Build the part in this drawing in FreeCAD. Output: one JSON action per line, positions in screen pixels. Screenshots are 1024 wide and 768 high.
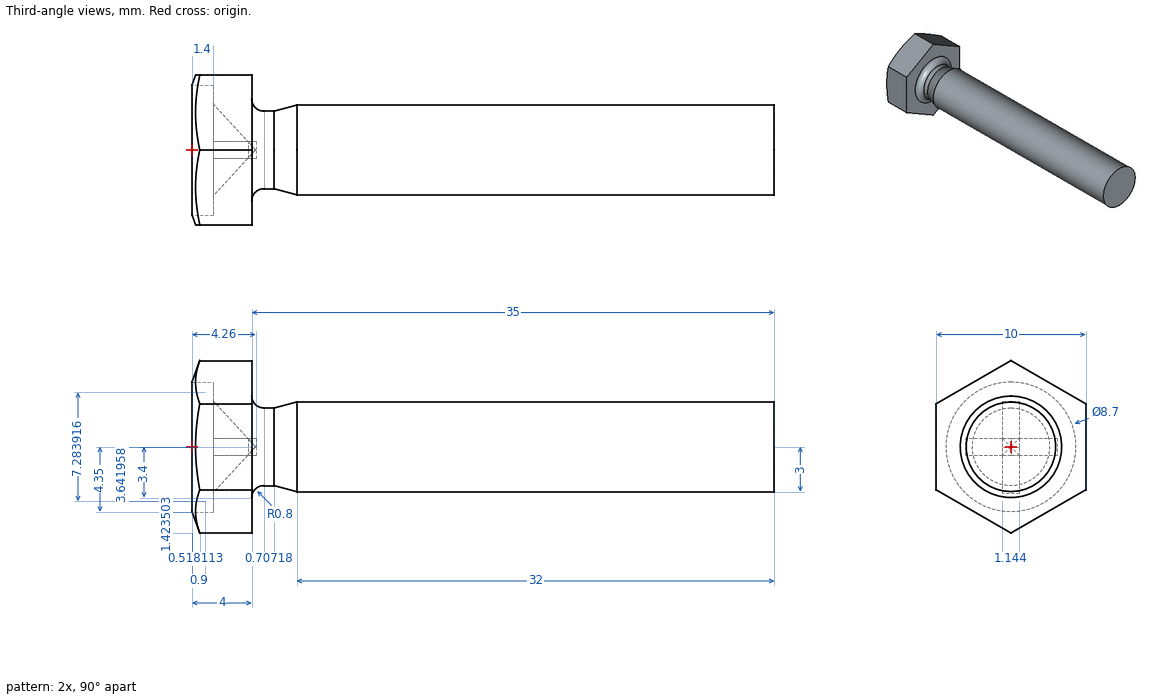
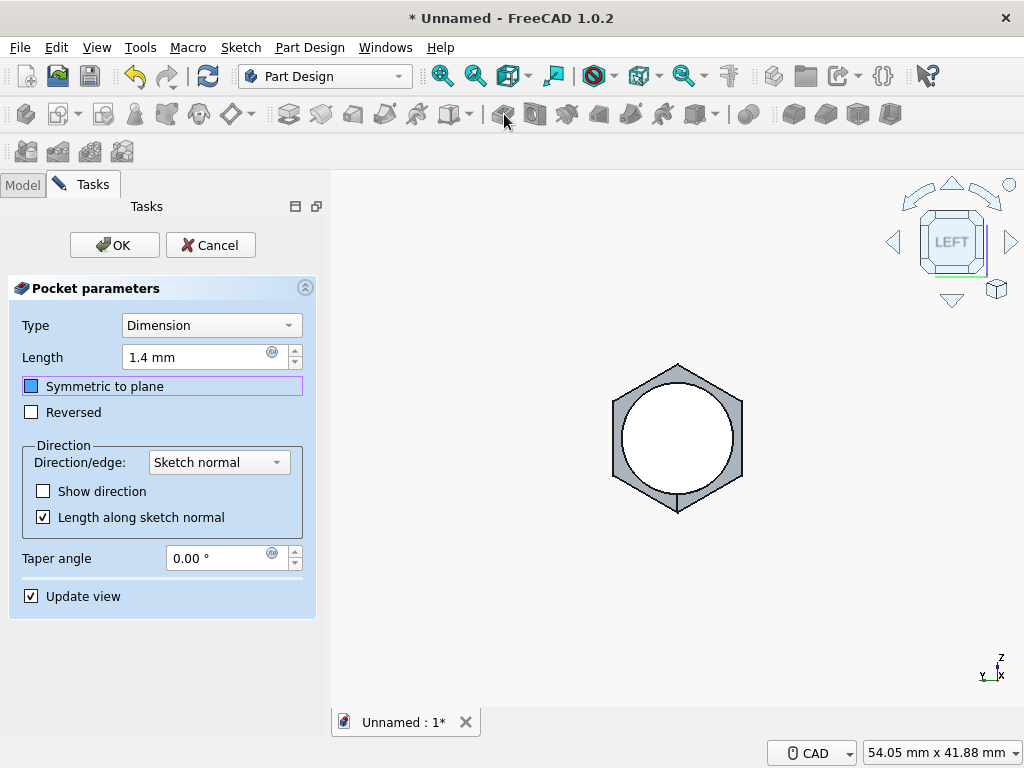
{"action": "left_click", "coordinate": [115, 245]}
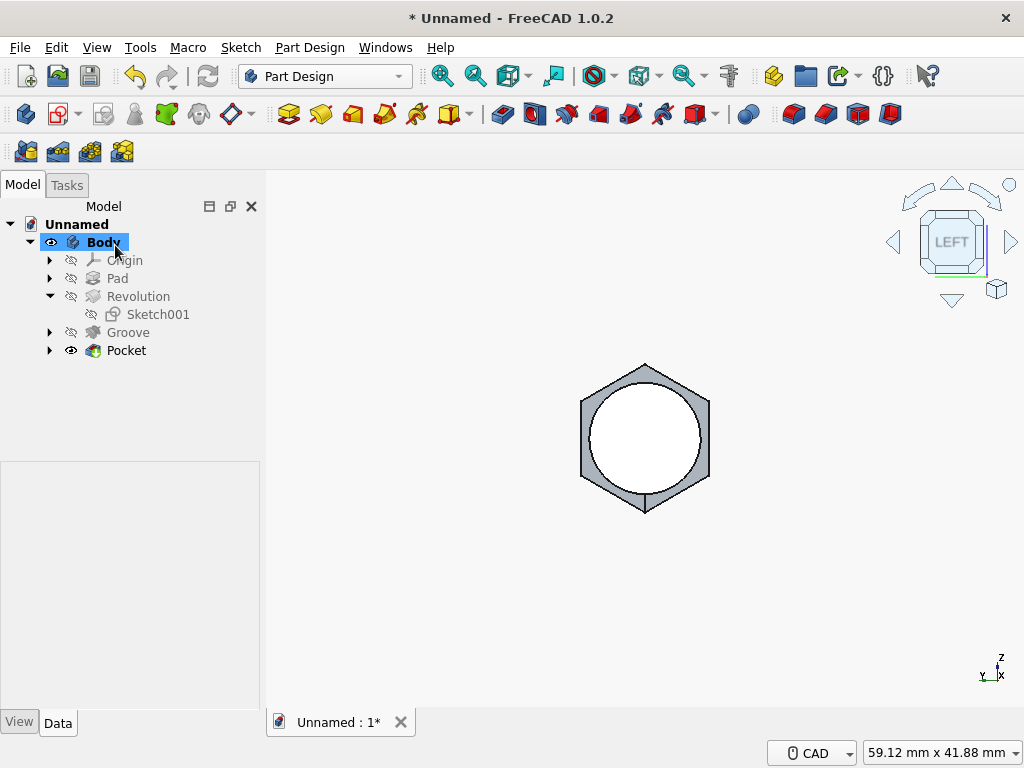
{"action": "left_click", "coordinate": [444, 76]}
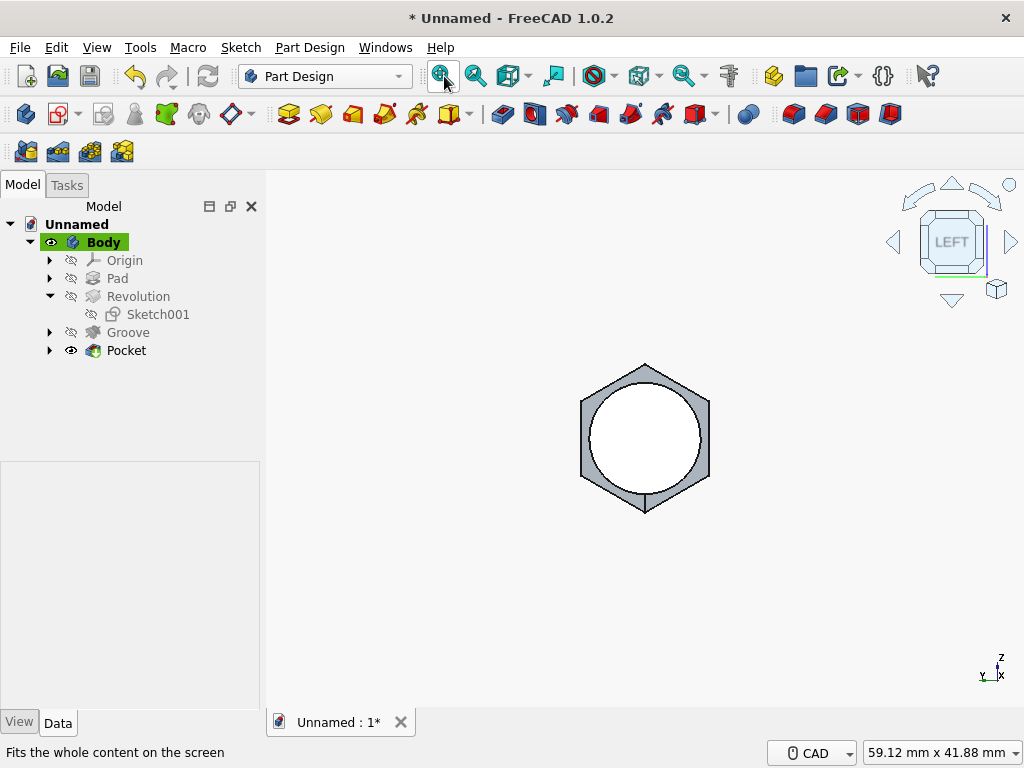
{"action": "left_click", "coordinate": [58, 114]}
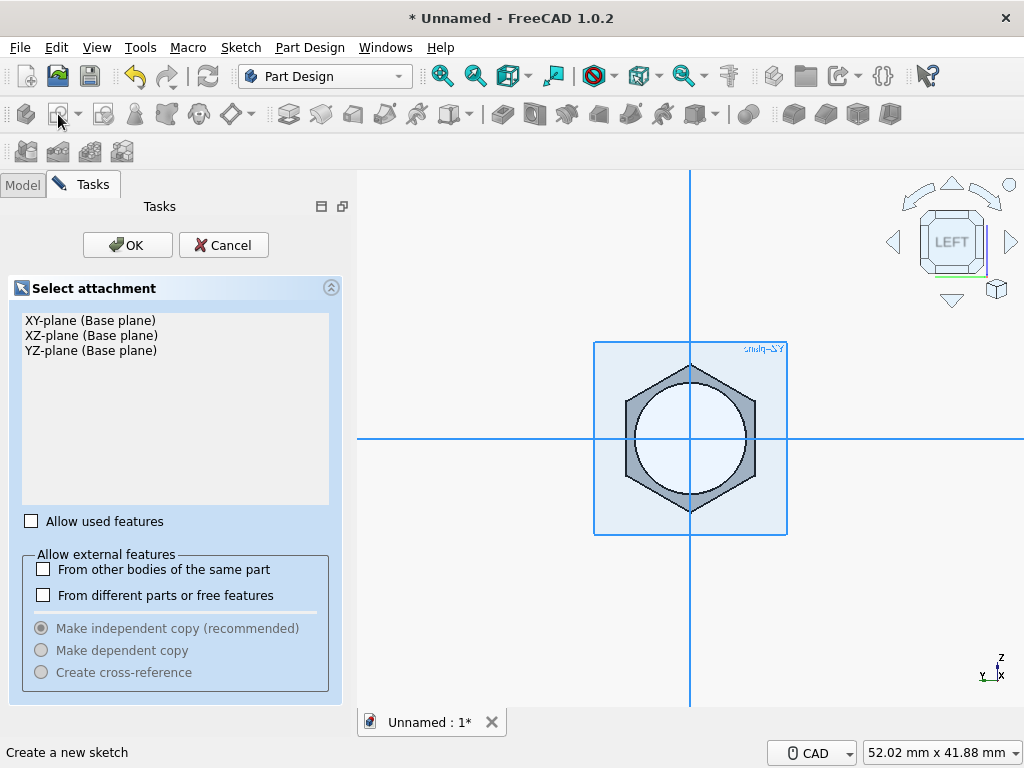
{"action": "left_click", "coordinate": [82, 336]}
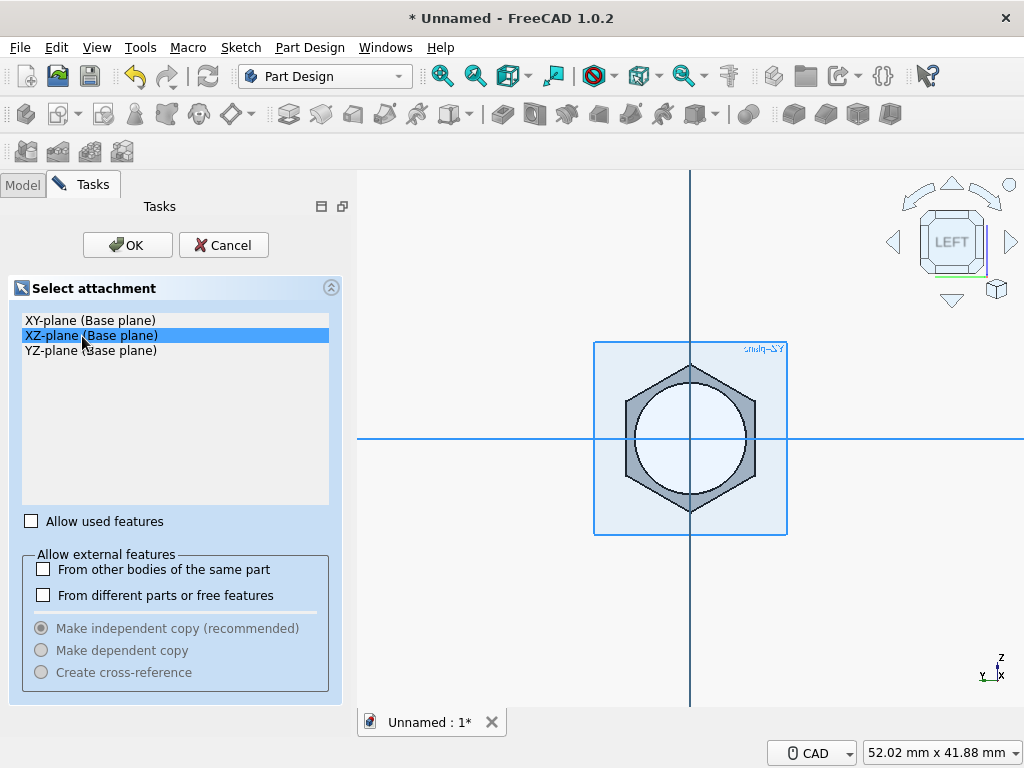
{"action": "left_click", "coordinate": [128, 245]}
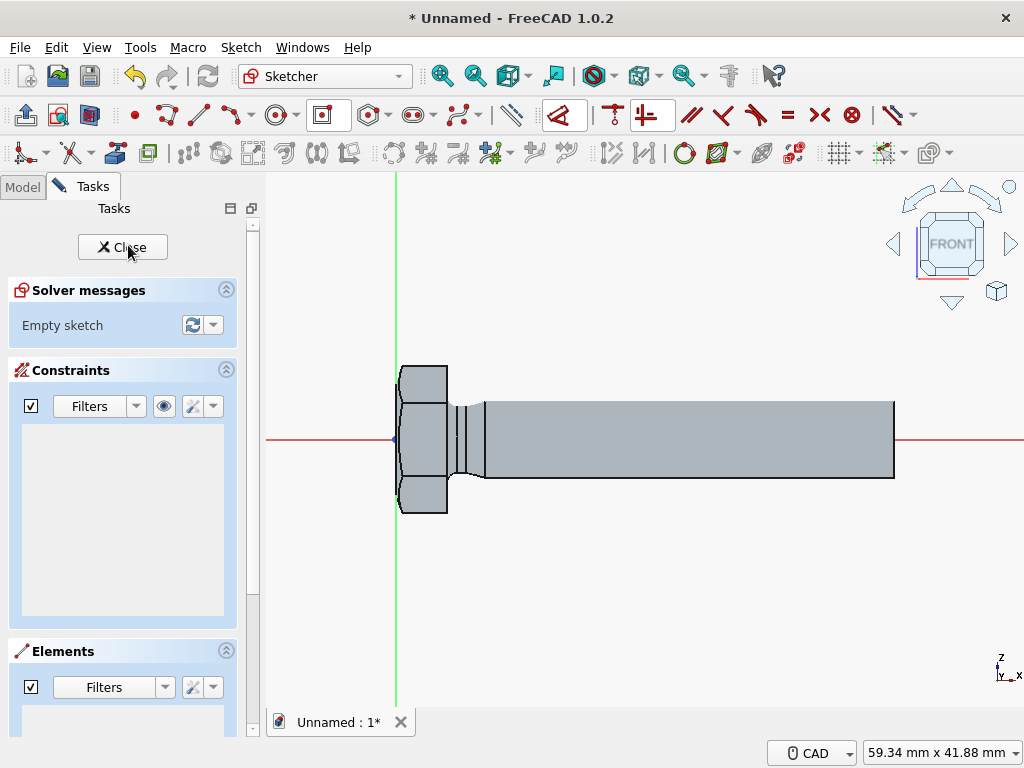
{"action": "left_click", "coordinate": [90, 116]}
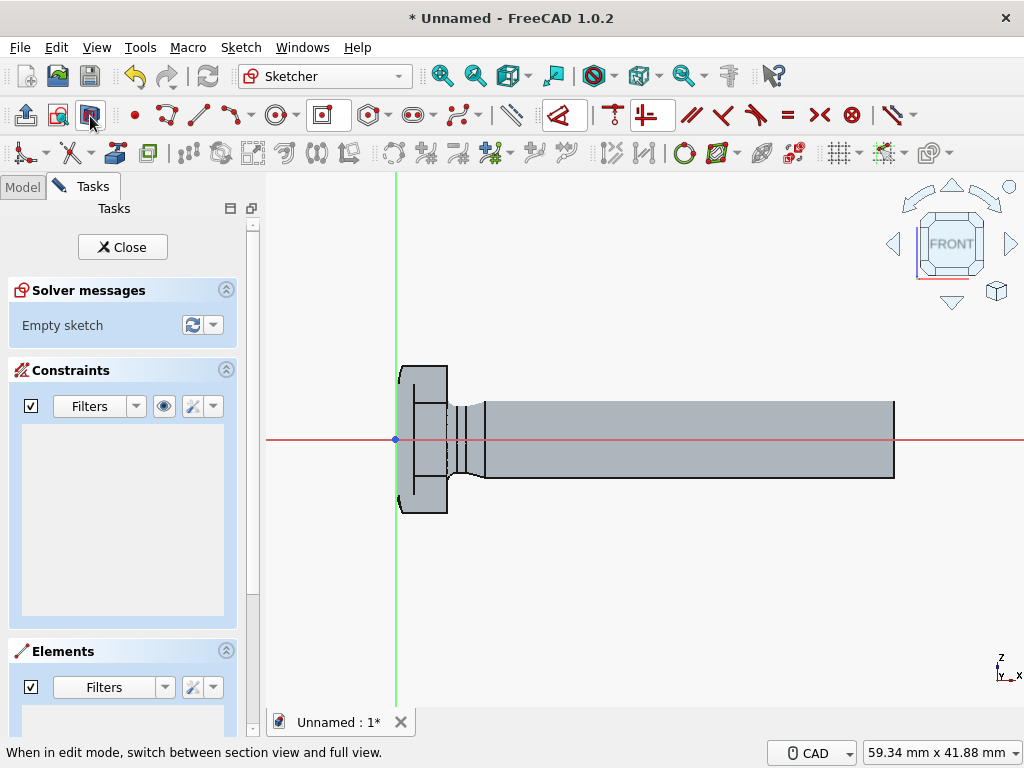
{"action": "scroll", "coordinate": [357, 440], "scroll_direction": "up", "scroll_amount": 6}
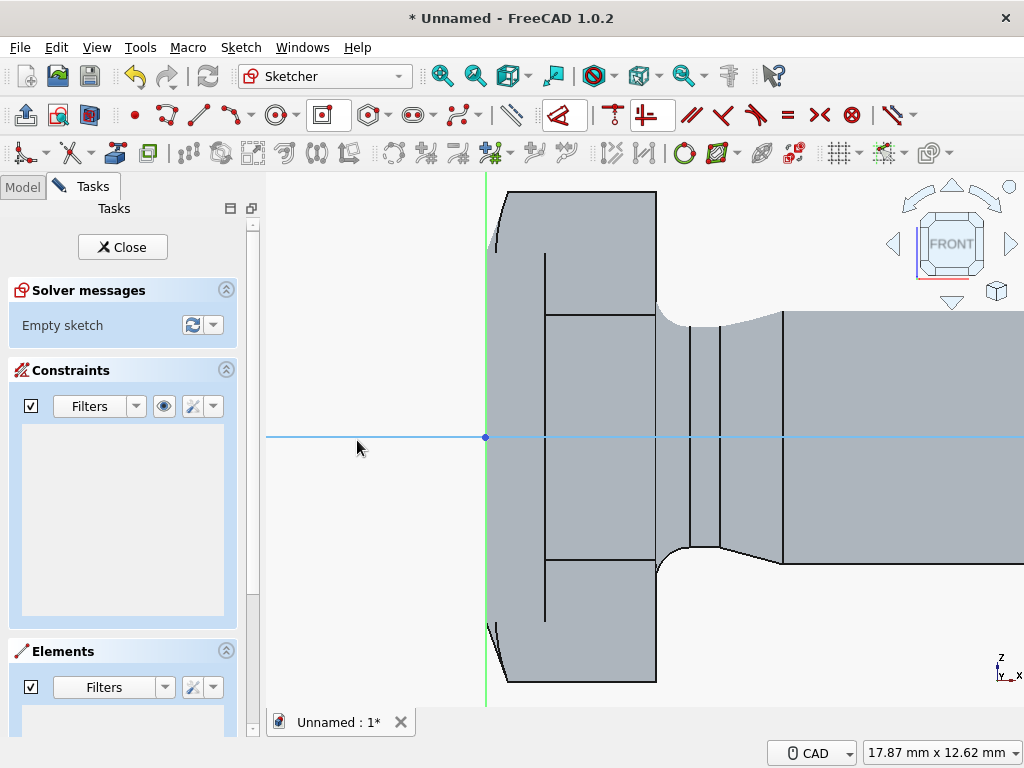
{"action": "left_click", "coordinate": [168, 116]}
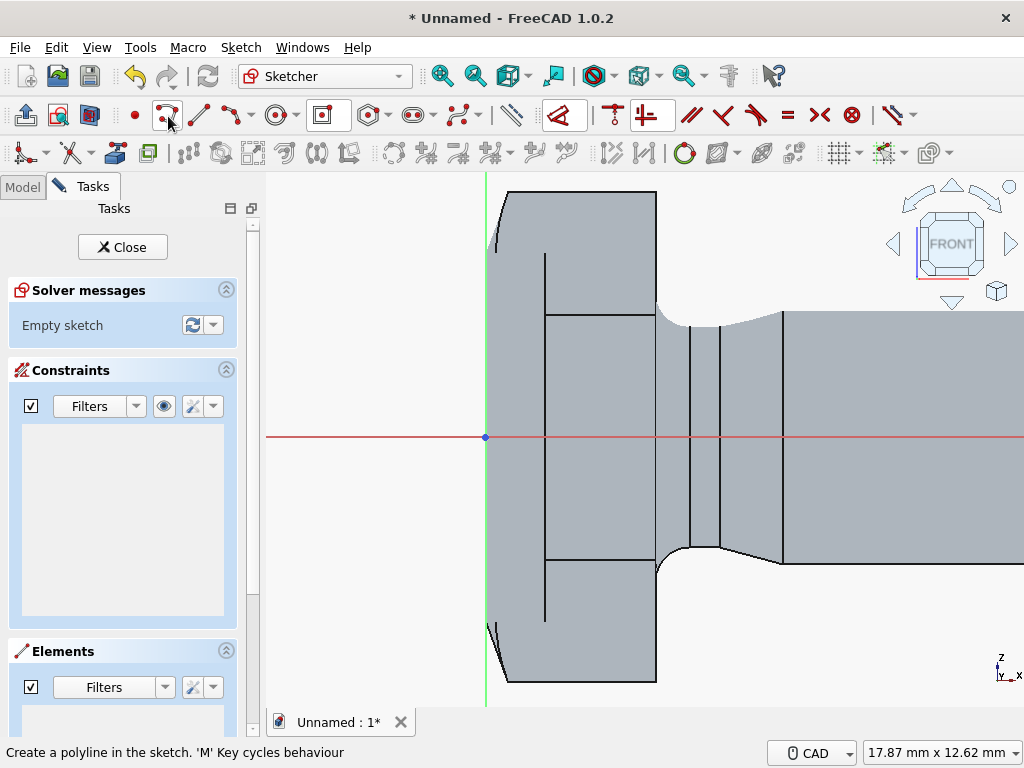
{"action": "left_click", "coordinate": [524, 592]}
{"action": "left_click", "coordinate": [524, 283]}
{"action": "left_click", "coordinate": [667, 437]}
{"action": "left_click", "coordinate": [524, 593]}
{"action": "key", "text": "Escape"}
{"action": "key", "text": "Escape"}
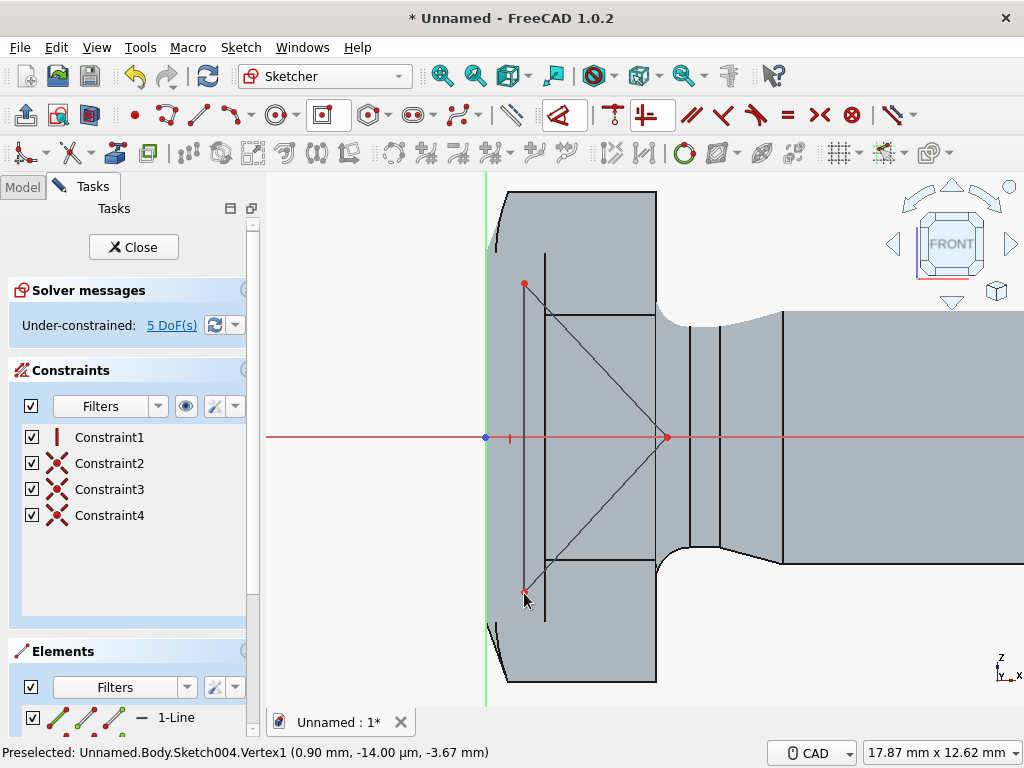
{"action": "left_click", "coordinate": [667, 437]}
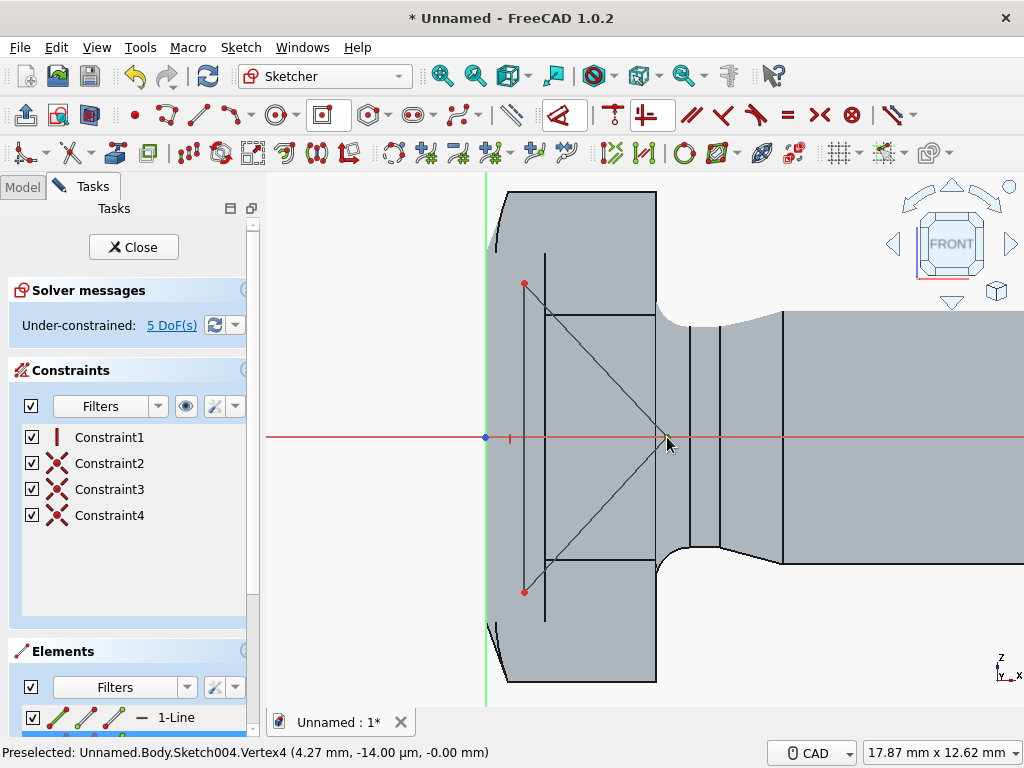
{"action": "left_click", "coordinate": [334, 437]}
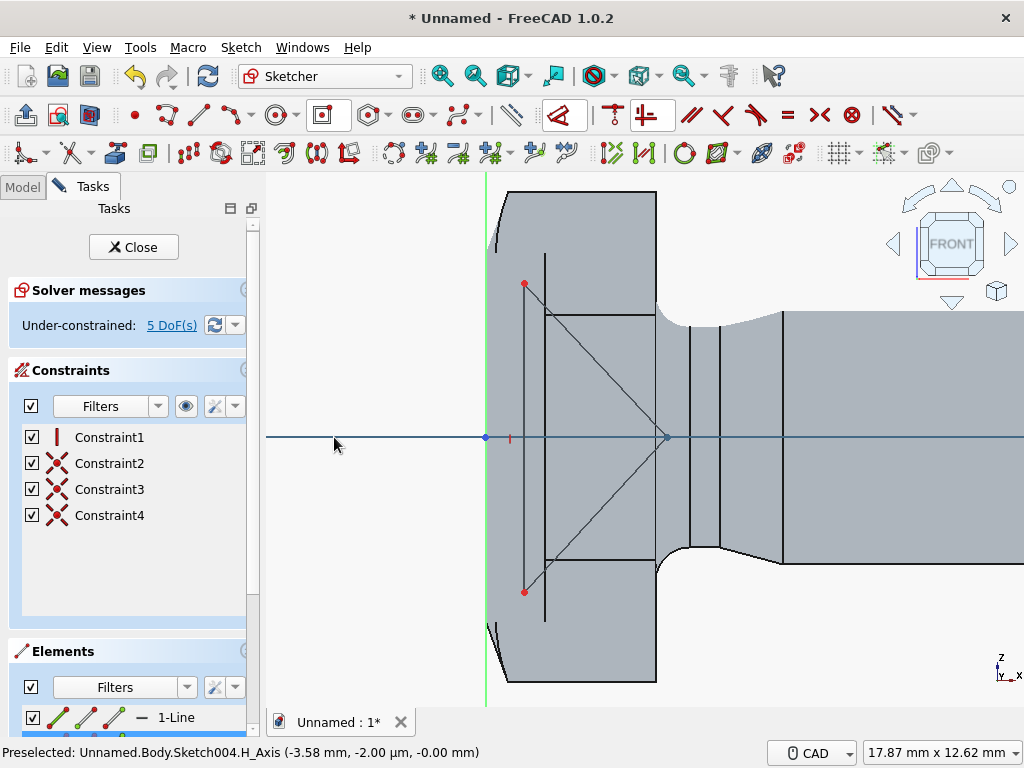
{"action": "left_click", "coordinate": [614, 116]}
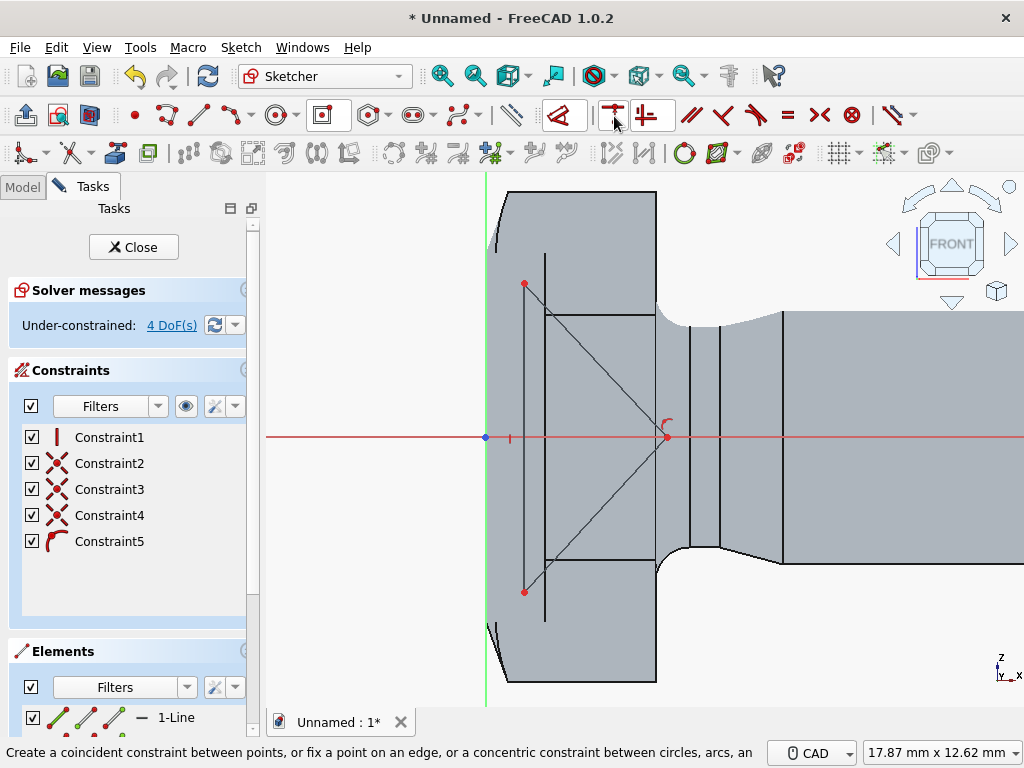
{"action": "left_click", "coordinate": [524, 593]}